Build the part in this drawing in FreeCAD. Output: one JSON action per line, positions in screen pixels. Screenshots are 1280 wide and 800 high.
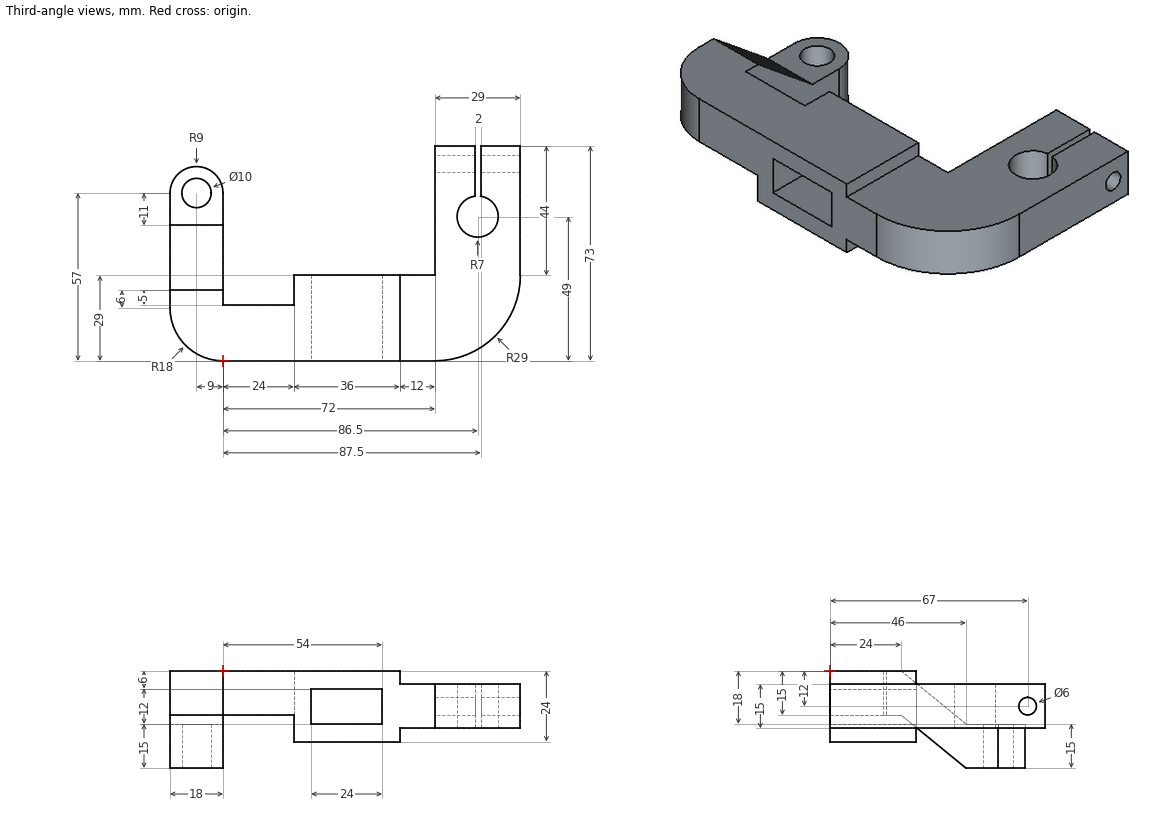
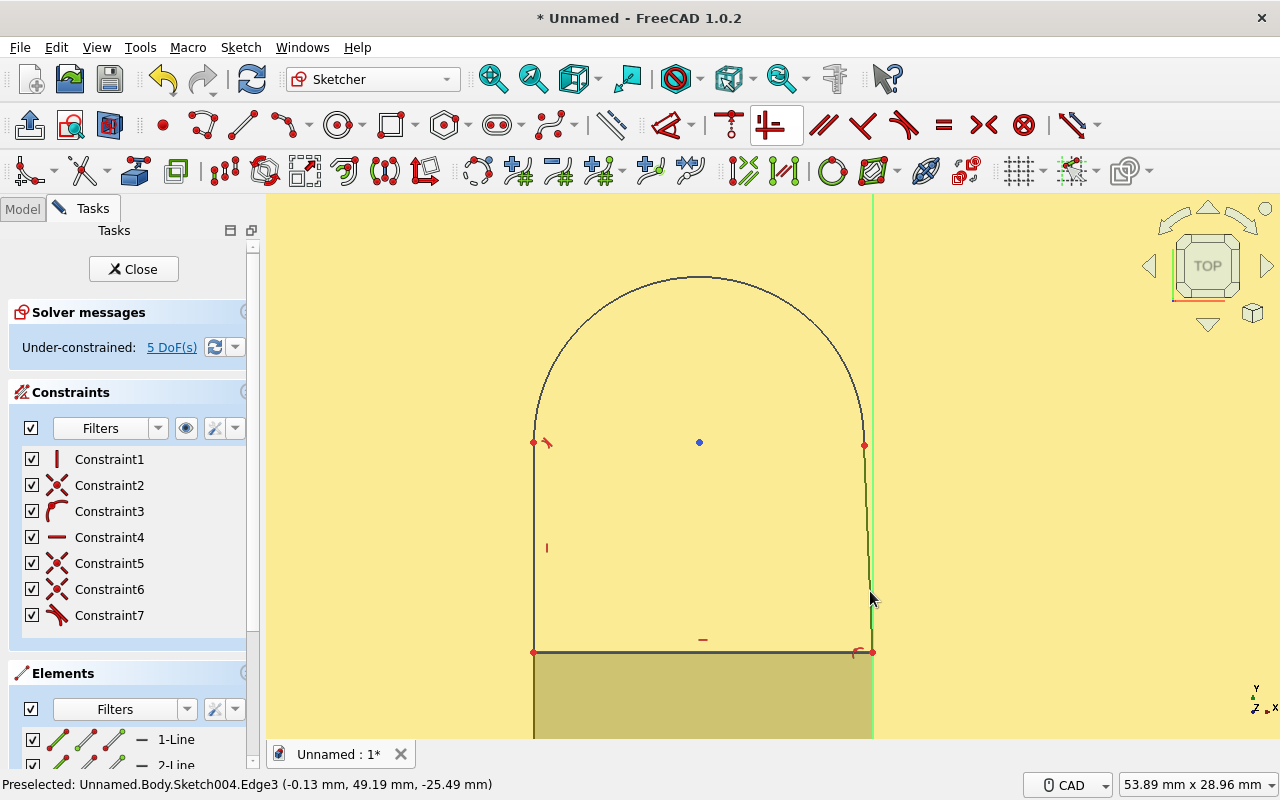
{"action": "left_click", "coordinate": [798, 310]}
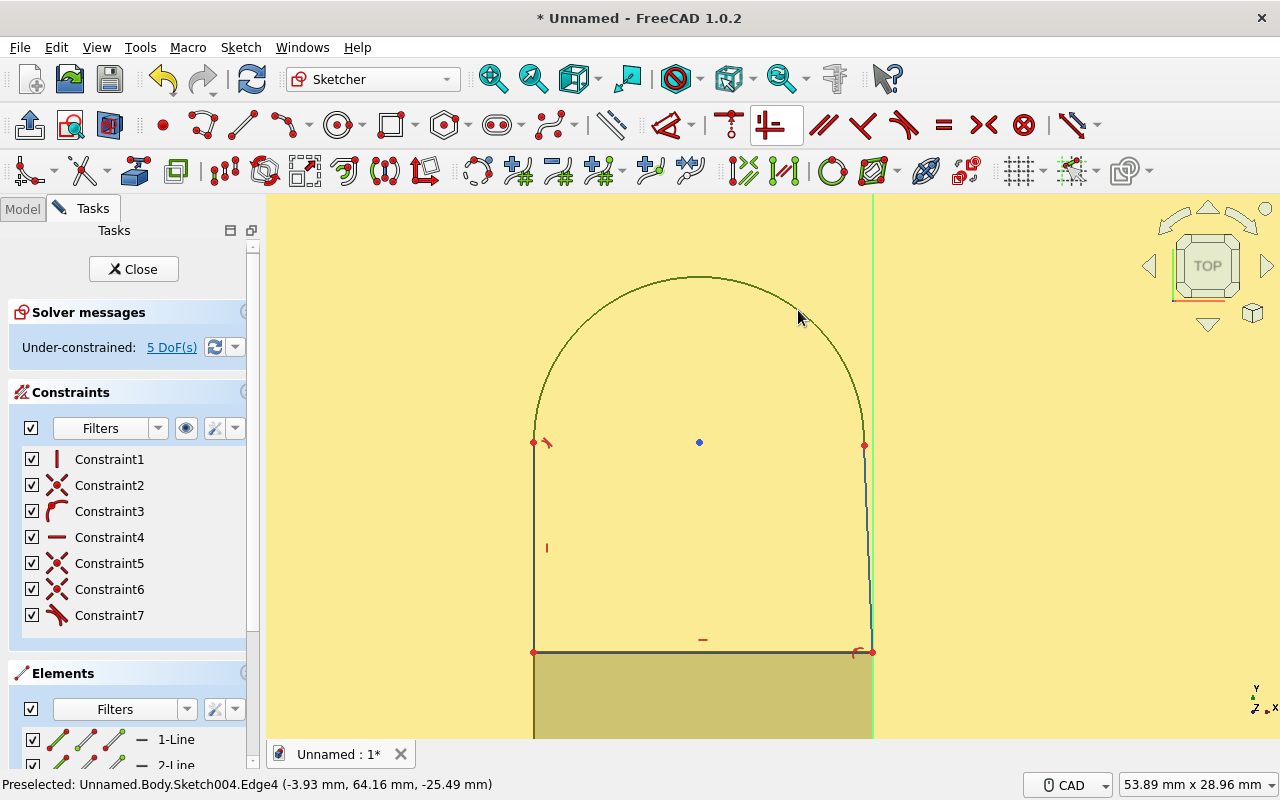
{"action": "key", "text": "t"}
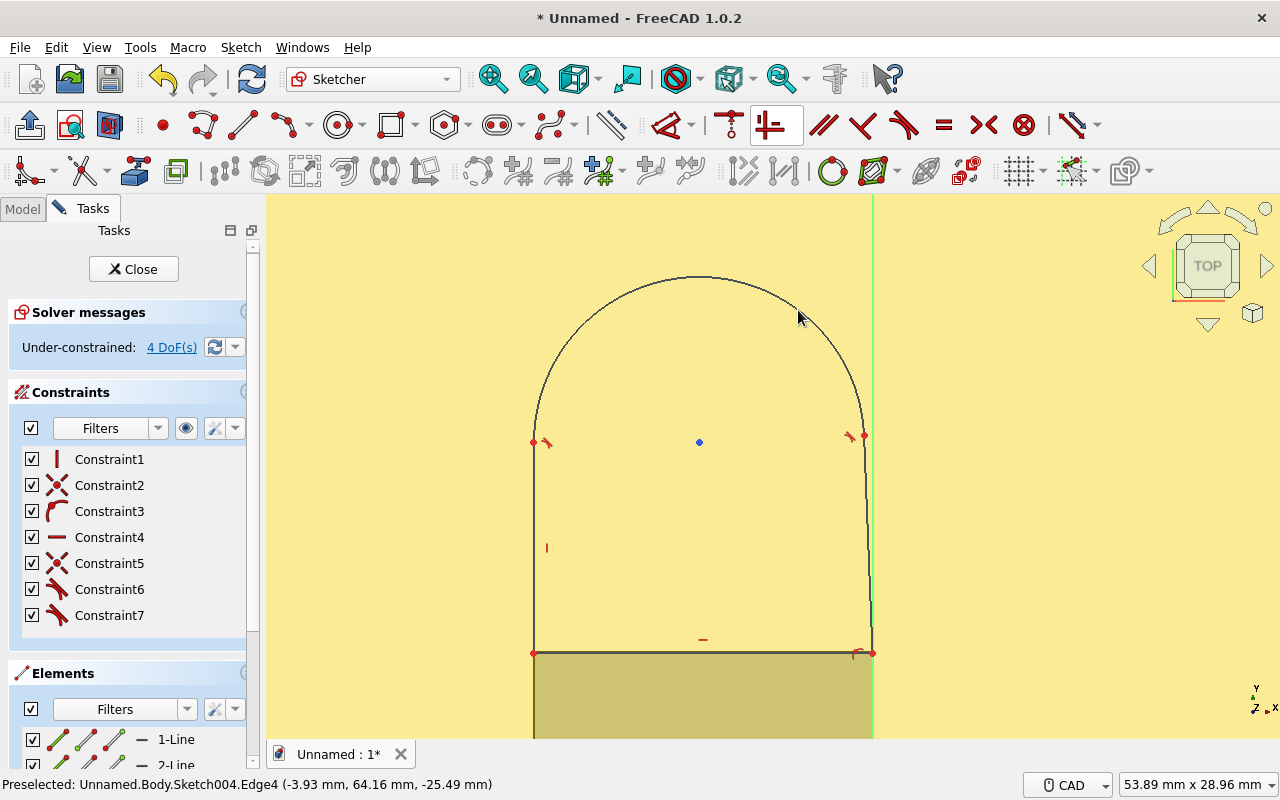
{"action": "left_click", "coordinate": [870, 588]}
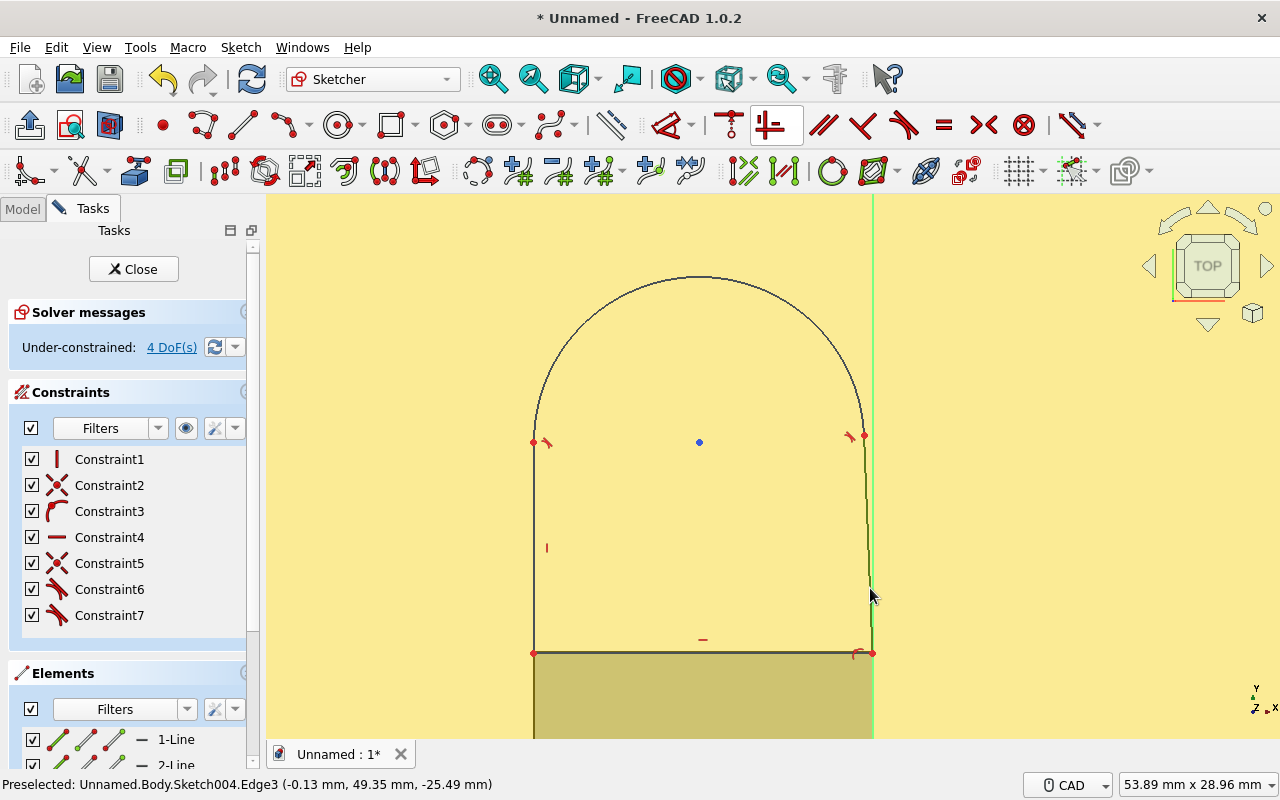
{"action": "key", "text": "v"}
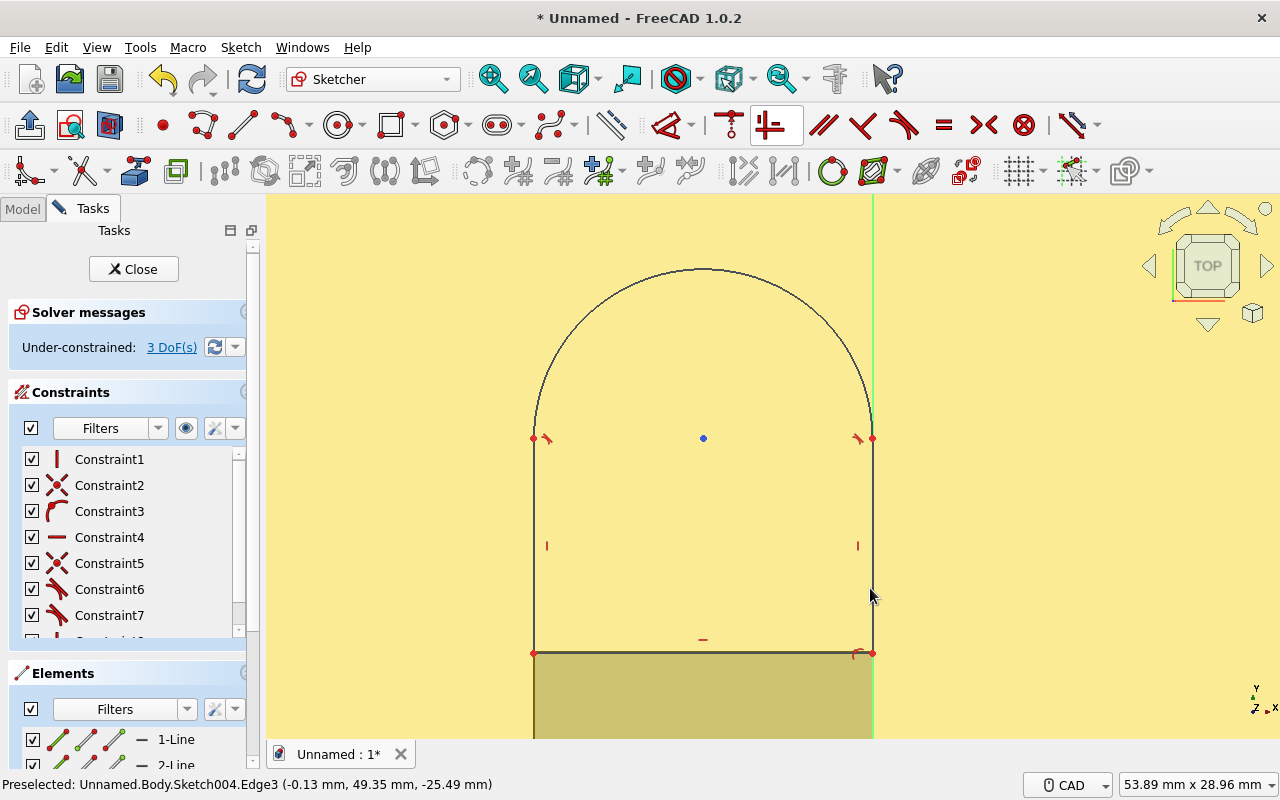
{"action": "left_click", "coordinate": [666, 126]}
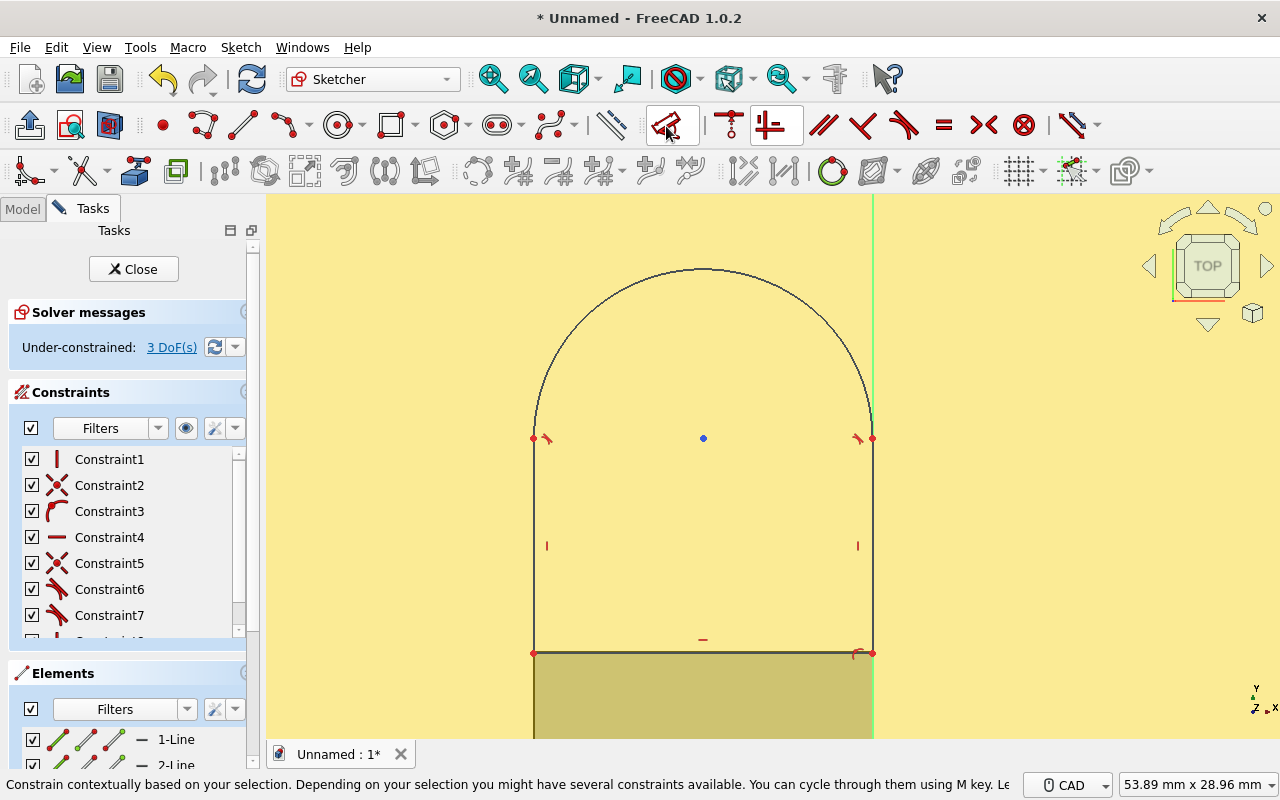
{"action": "left_click", "coordinate": [803, 302]}
{"action": "left_click", "coordinate": [822, 276]}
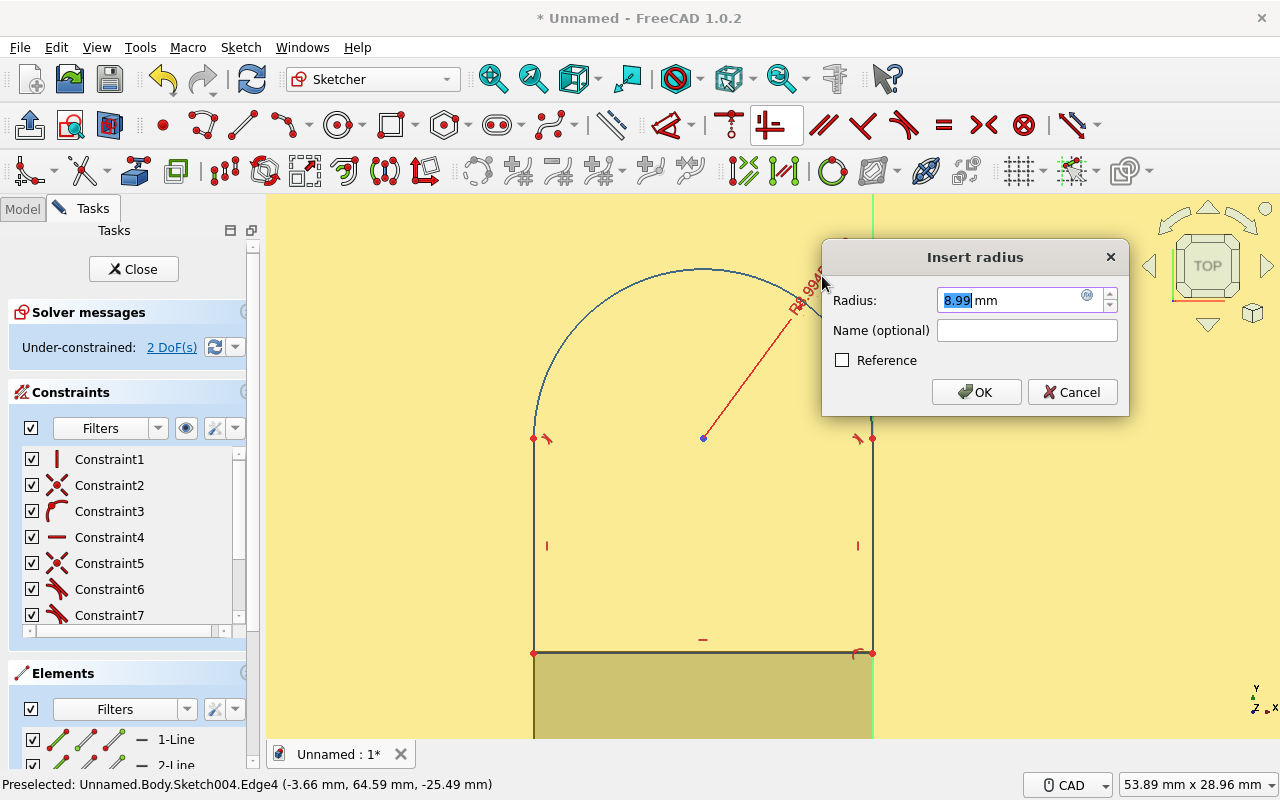
{"action": "type", "text": "9"}
{"action": "key", "text": "Return"}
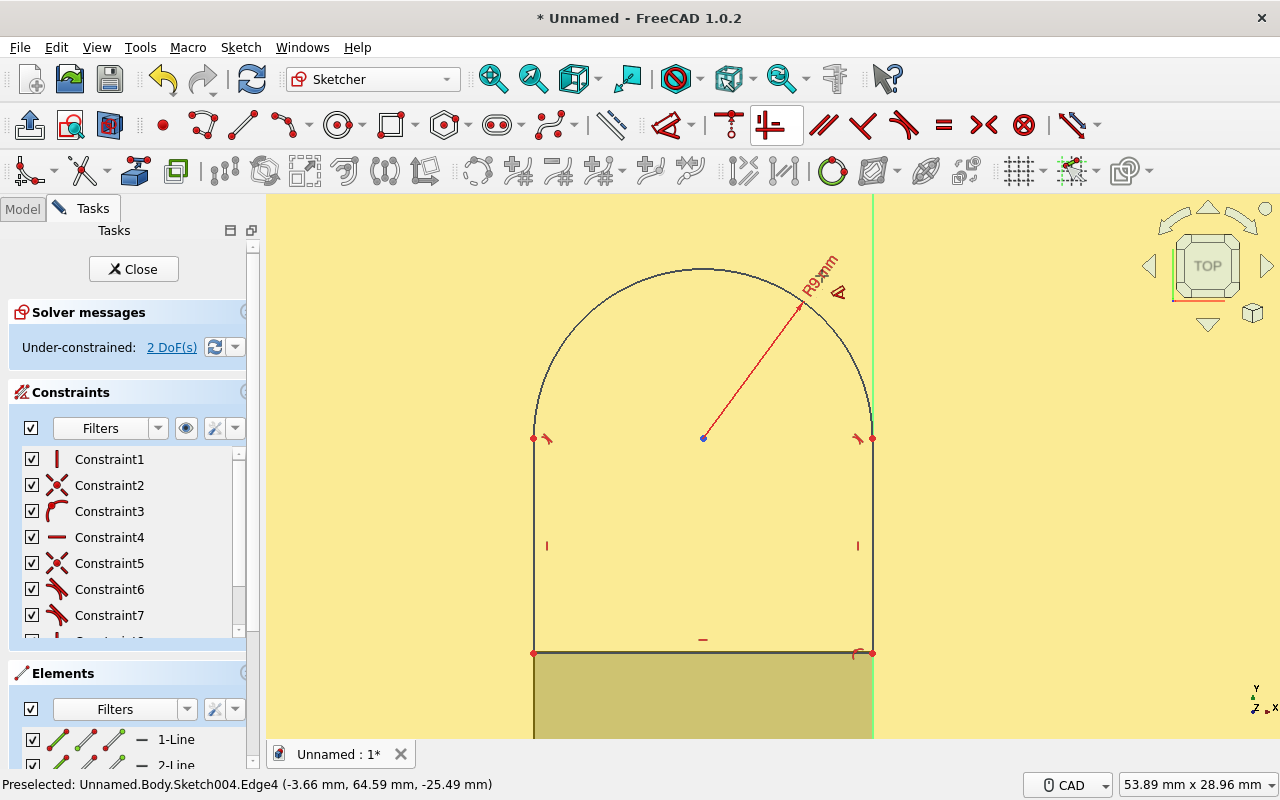
{"action": "left_click", "coordinate": [534, 503]}
{"action": "left_click", "coordinate": [500, 546]}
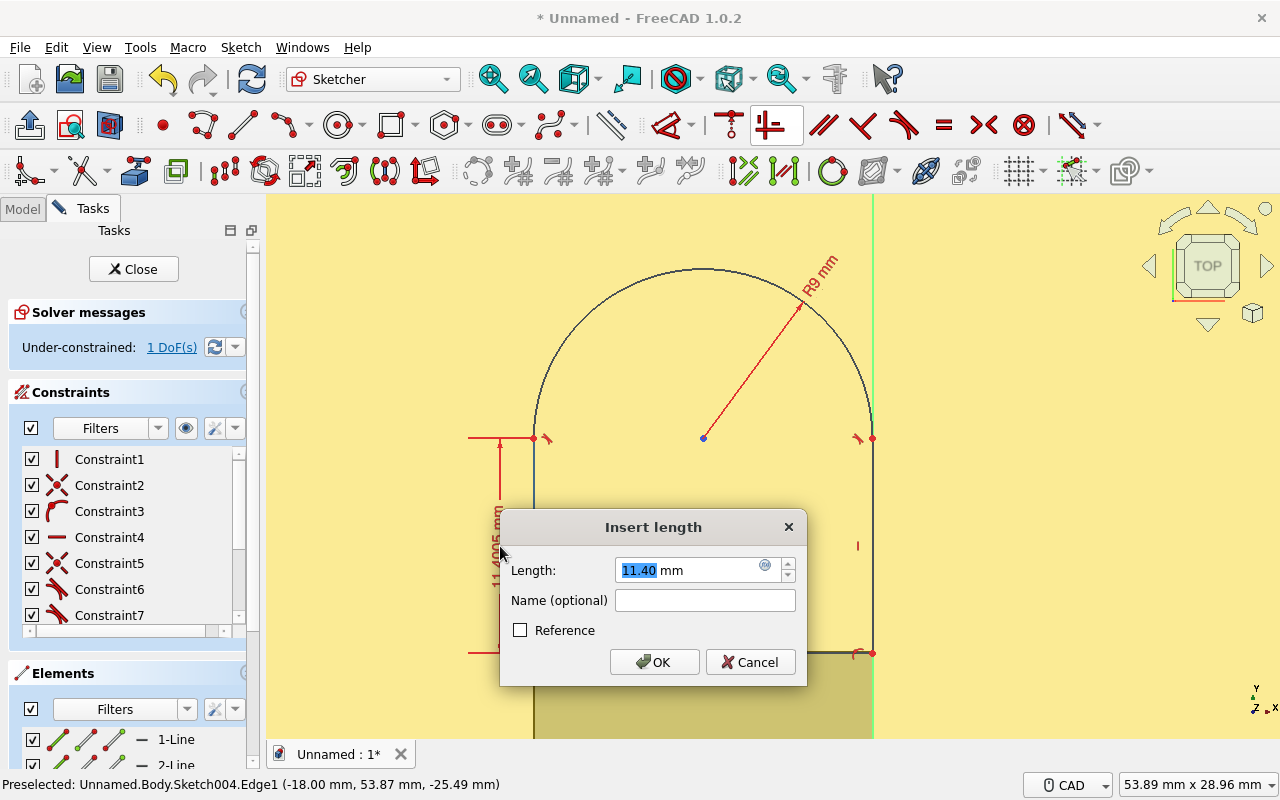
{"action": "type", "text": "11"}
{"action": "key", "text": "Return"}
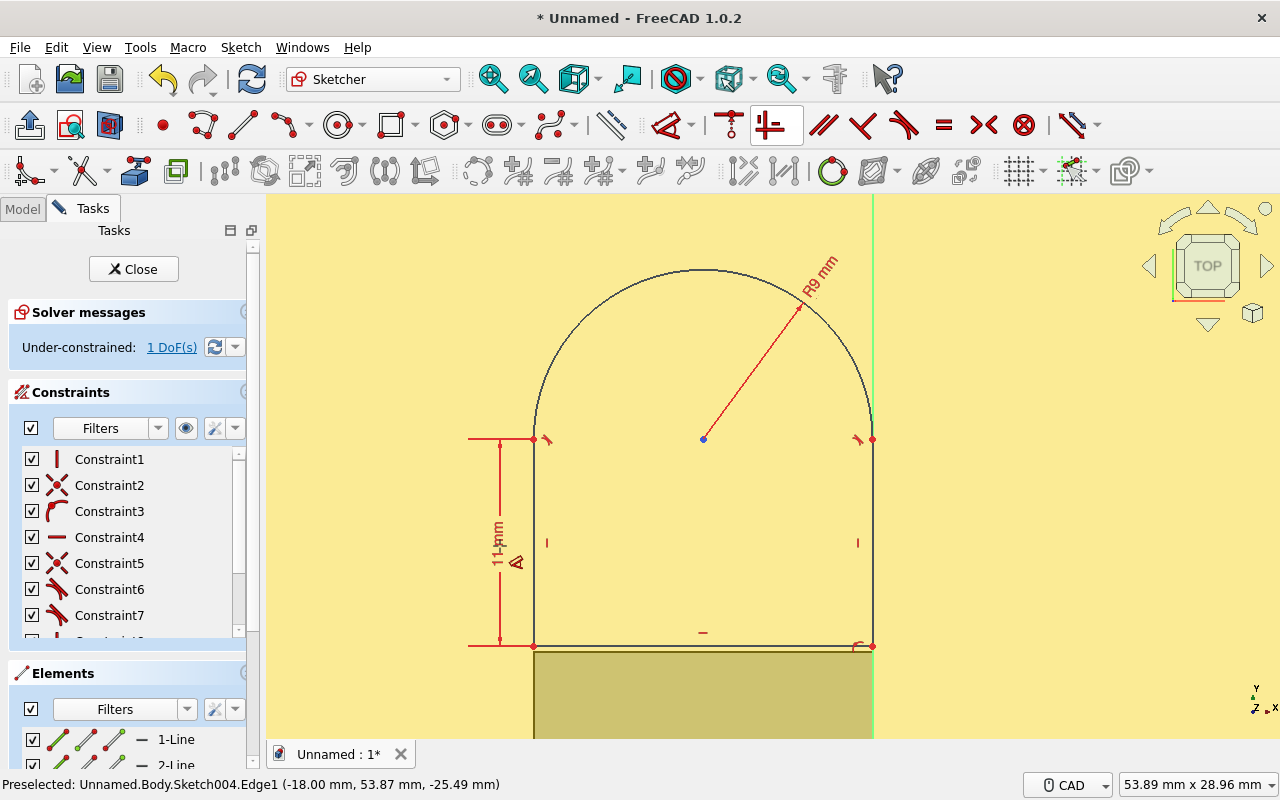
{"action": "left_click", "coordinate": [534, 439]}
{"action": "left_click", "coordinate": [907, 575]}